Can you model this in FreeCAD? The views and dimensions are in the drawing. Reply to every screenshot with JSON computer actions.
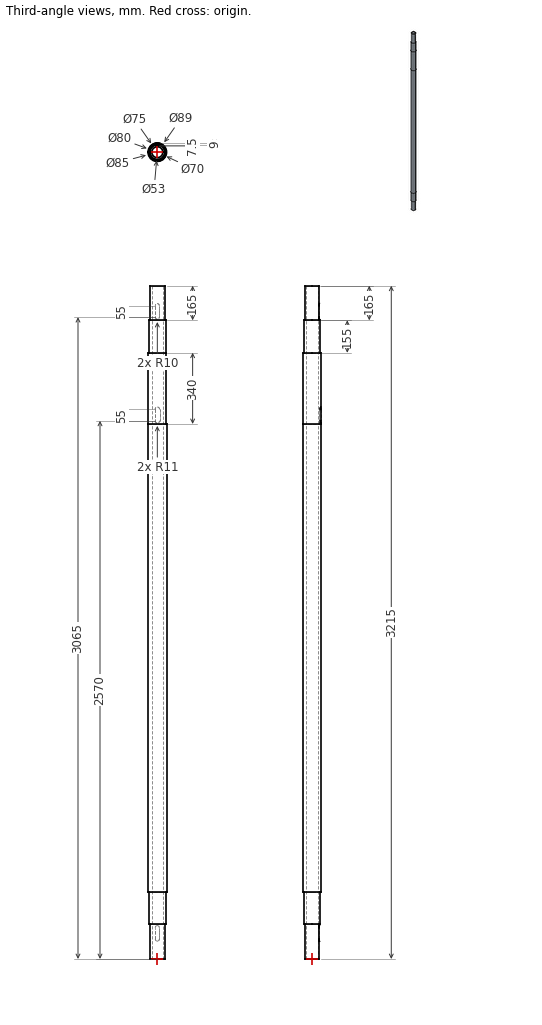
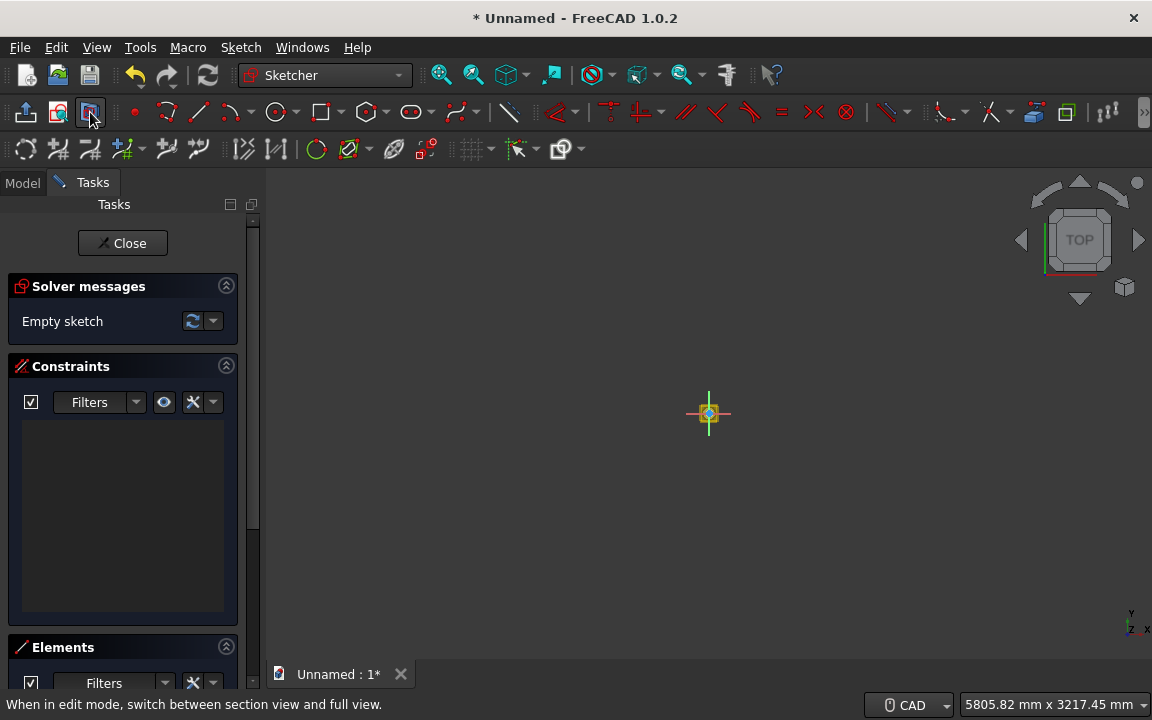
{"action": "scroll", "coordinate": [713, 414], "scroll_direction": "up", "scroll_amount": 15}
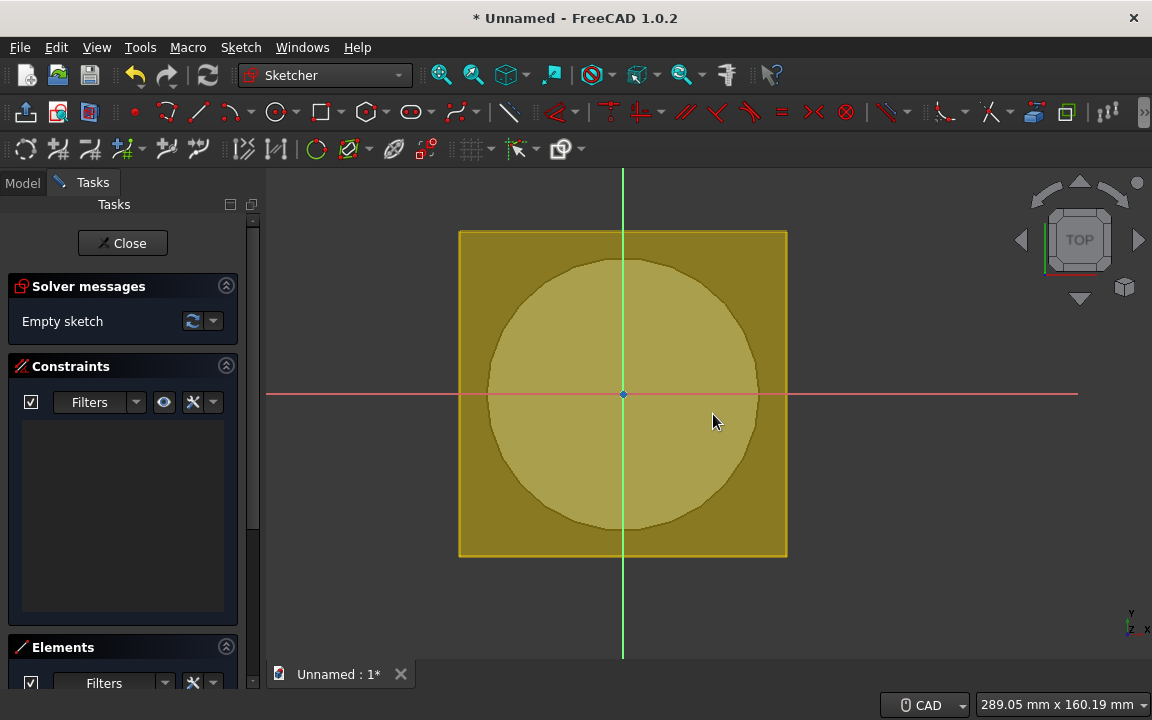
{"action": "left_click", "coordinate": [276, 112]}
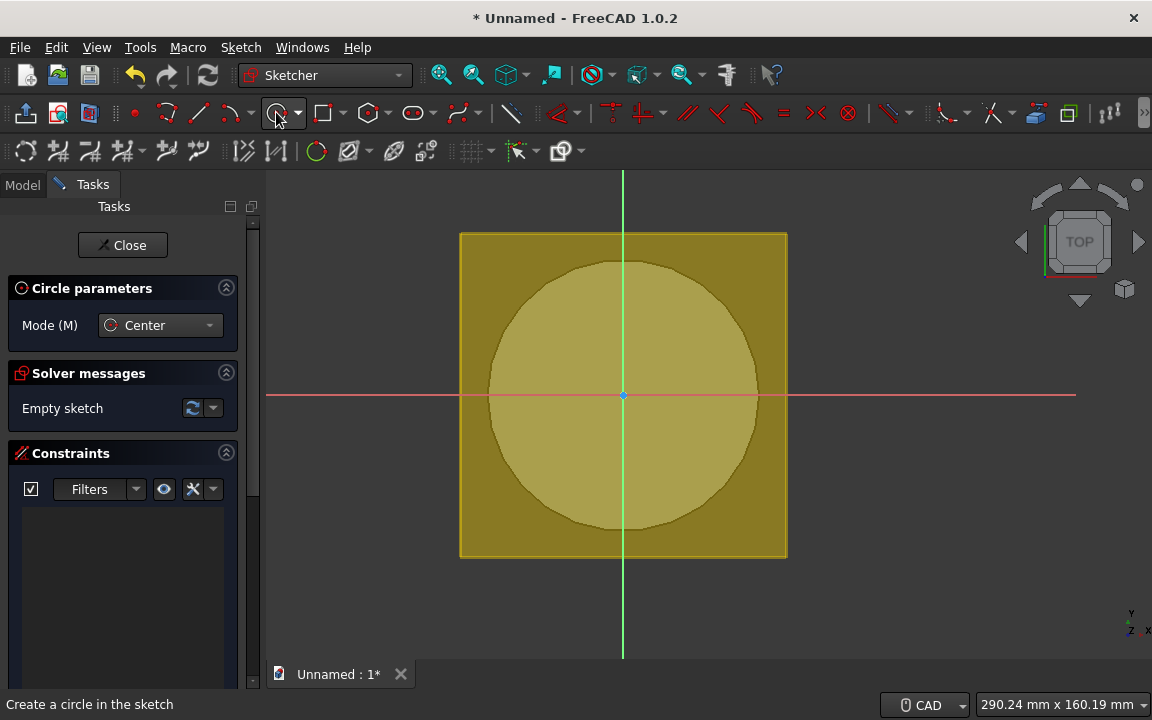
{"action": "left_click", "coordinate": [623, 395]}
{"action": "mouse_move", "coordinate": [719, 299]}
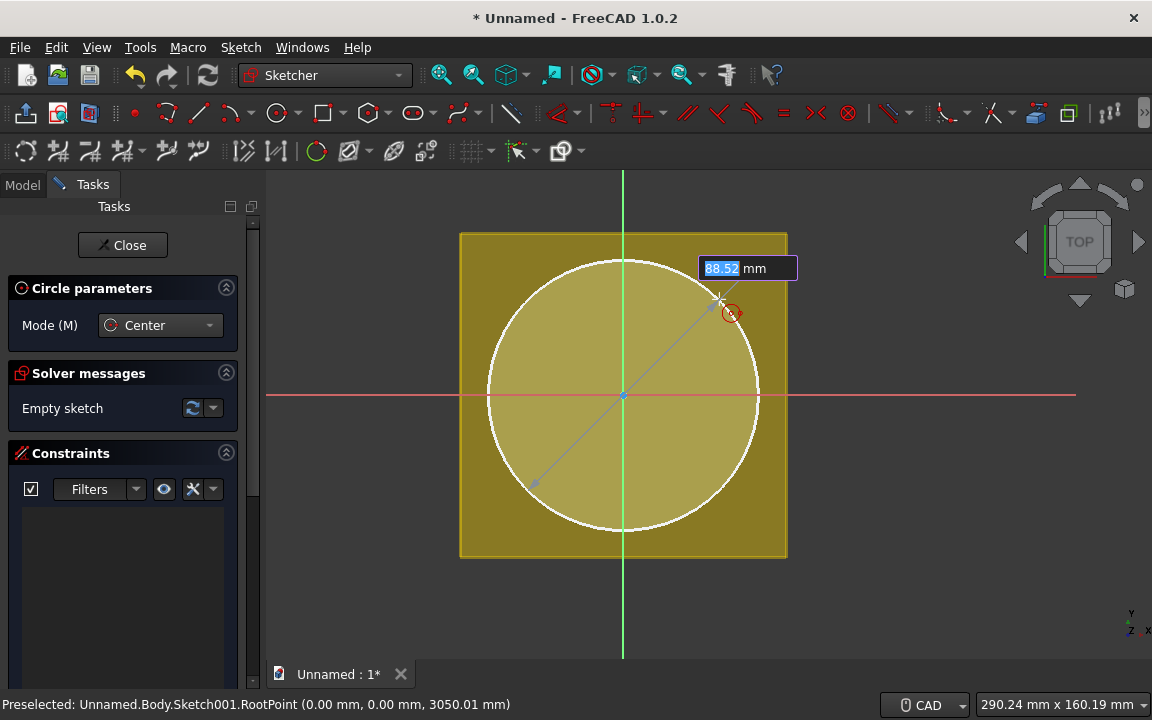
{"action": "type", "text": "89"}
{"action": "key", "text": "Return"}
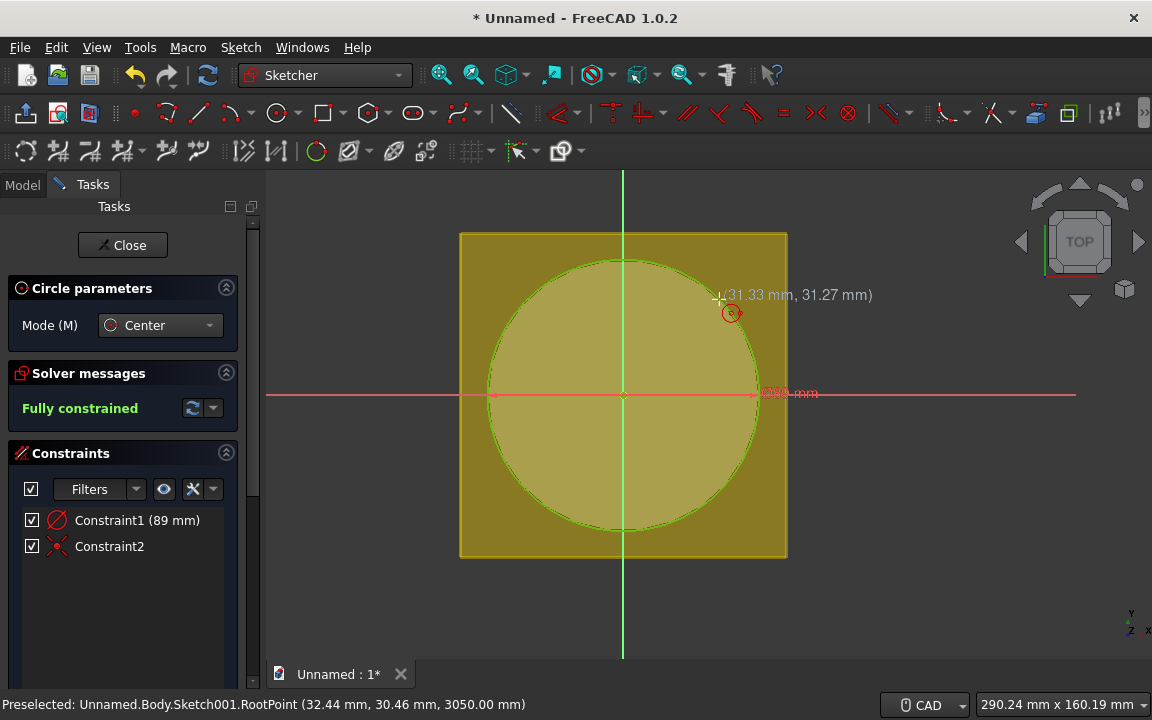
{"action": "left_click", "coordinate": [623, 395]}
{"action": "mouse_move", "coordinate": [704, 315]}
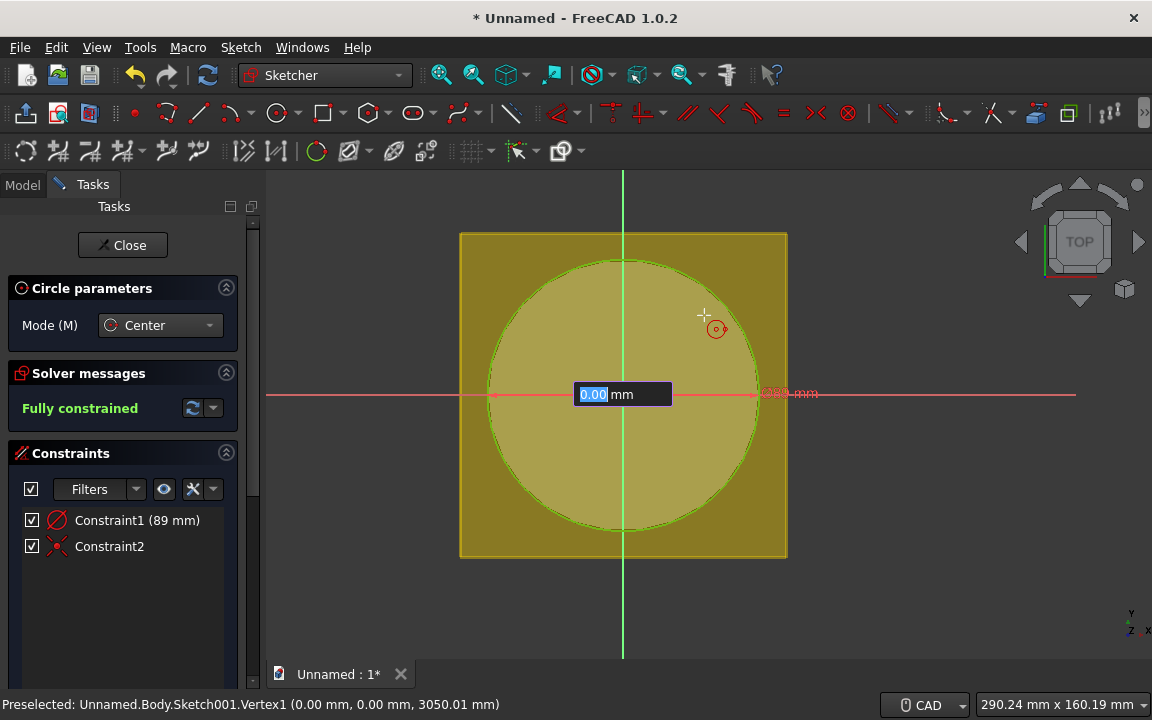
{"action": "type", "text": "75"}
{"action": "key", "text": "Return"}
{"action": "key", "text": "Escape"}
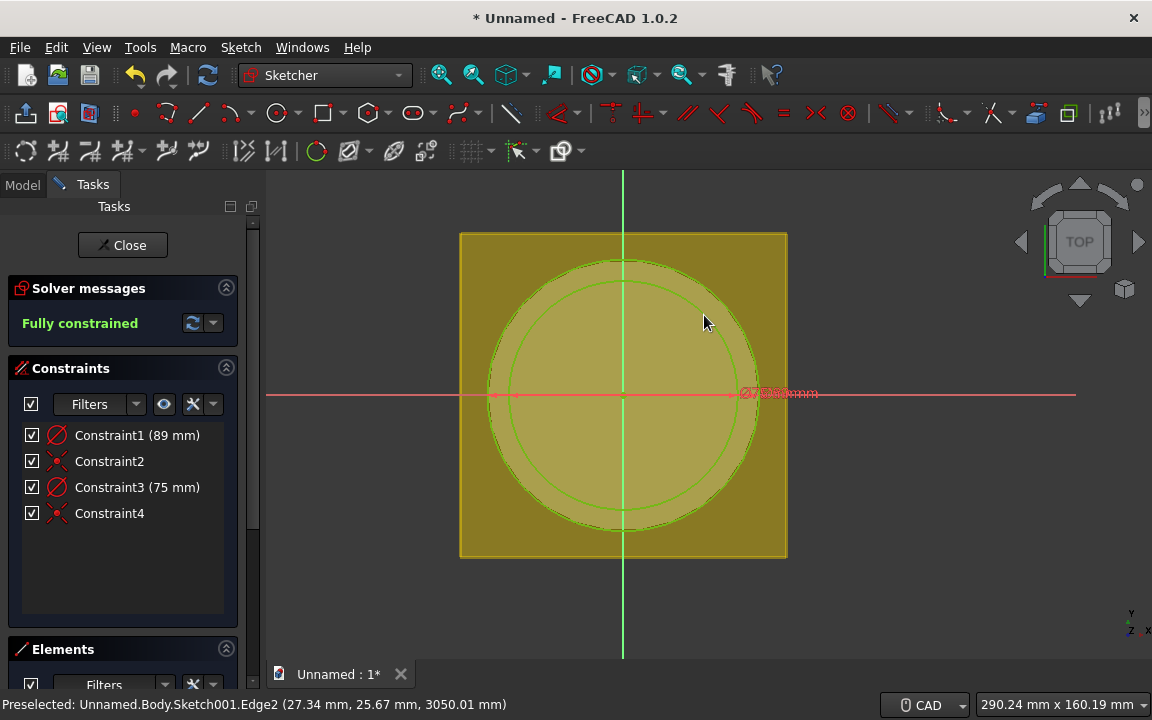
{"action": "left_click", "coordinate": [123, 245]}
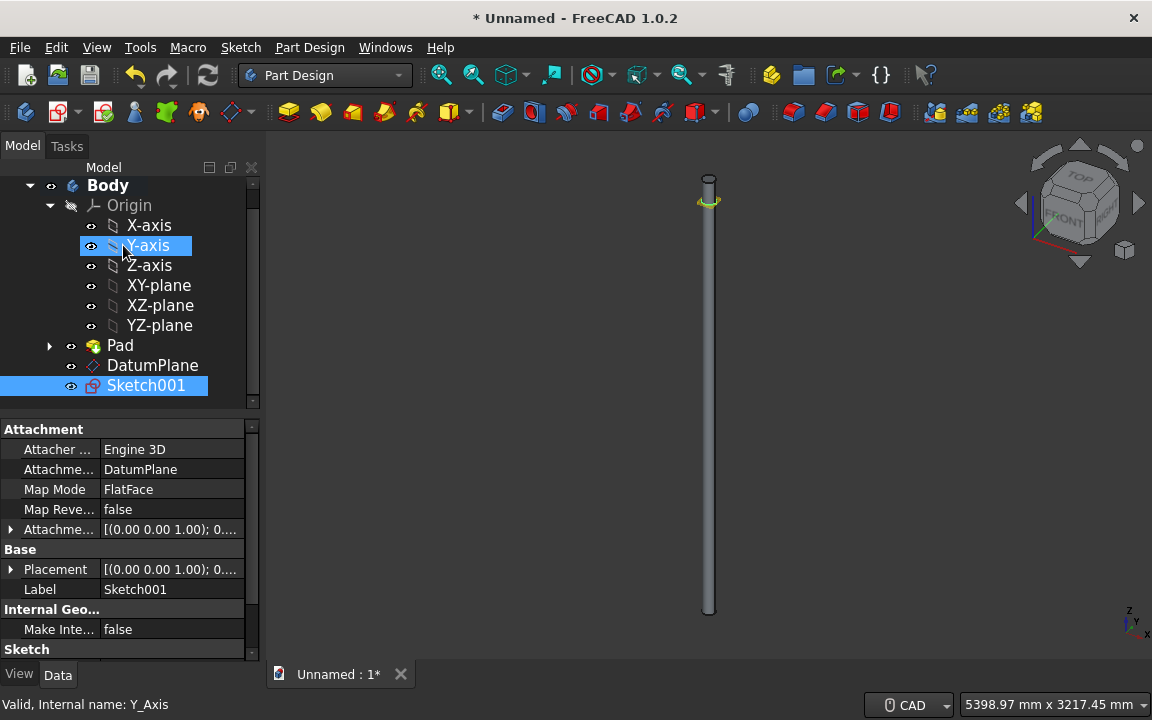
{"action": "left_click", "coordinate": [504, 112]}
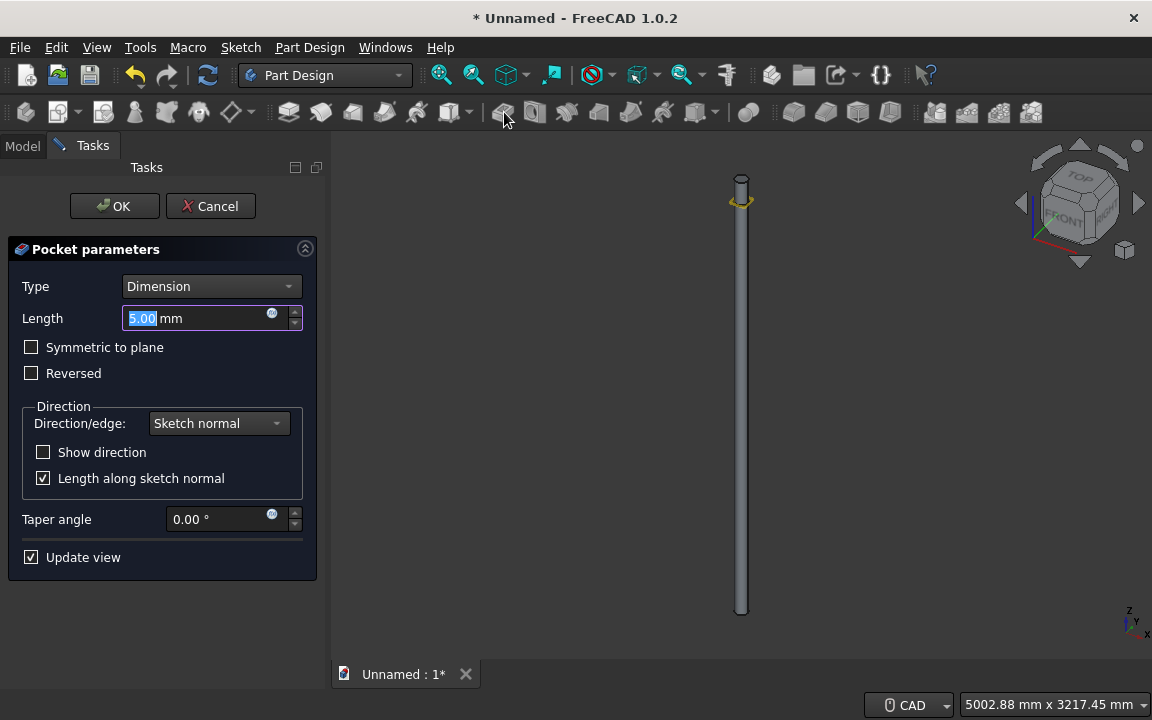
{"action": "type", "text": "165"}
{"action": "key", "text": "Tab"}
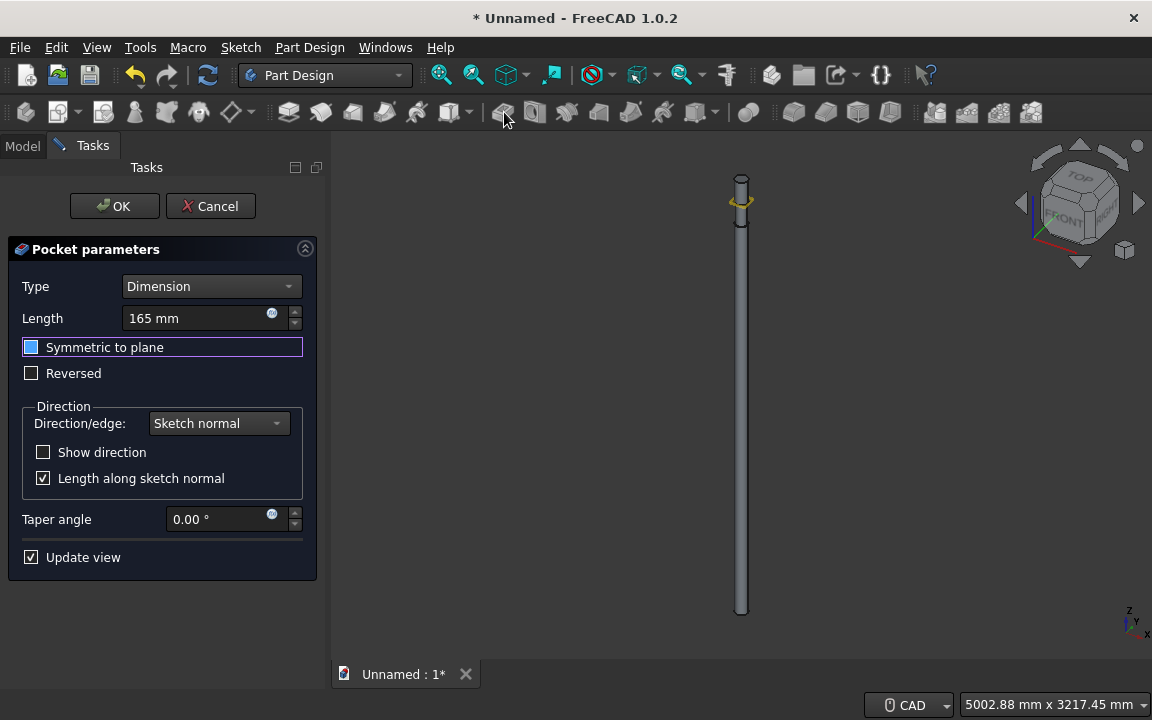
{"action": "left_click", "coordinate": [30, 373]}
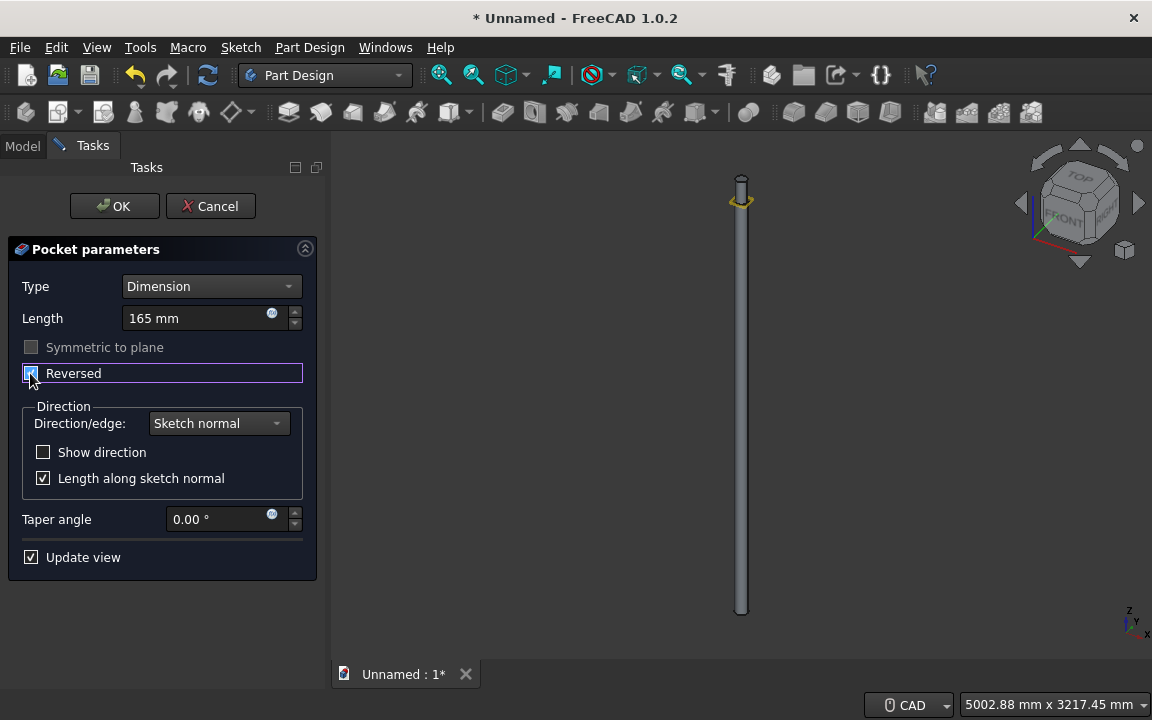
{"action": "left_click", "coordinate": [115, 206]}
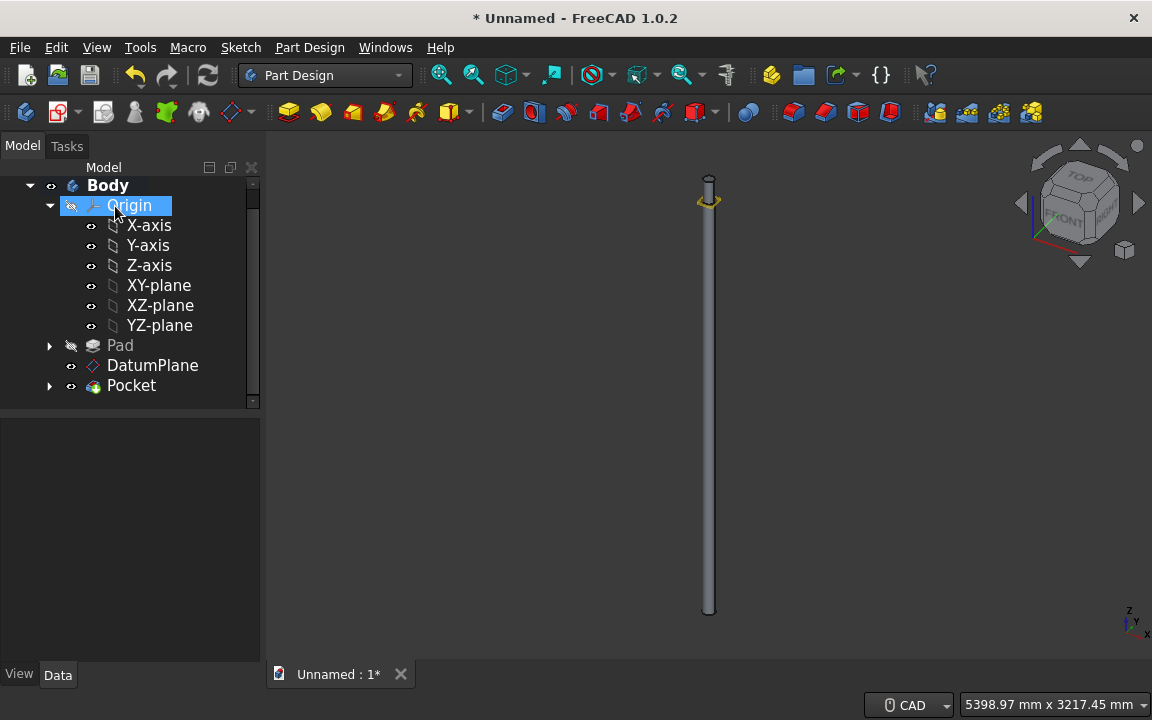
{"action": "left_click", "coordinate": [116, 366]}
{"action": "key", "text": "space"}